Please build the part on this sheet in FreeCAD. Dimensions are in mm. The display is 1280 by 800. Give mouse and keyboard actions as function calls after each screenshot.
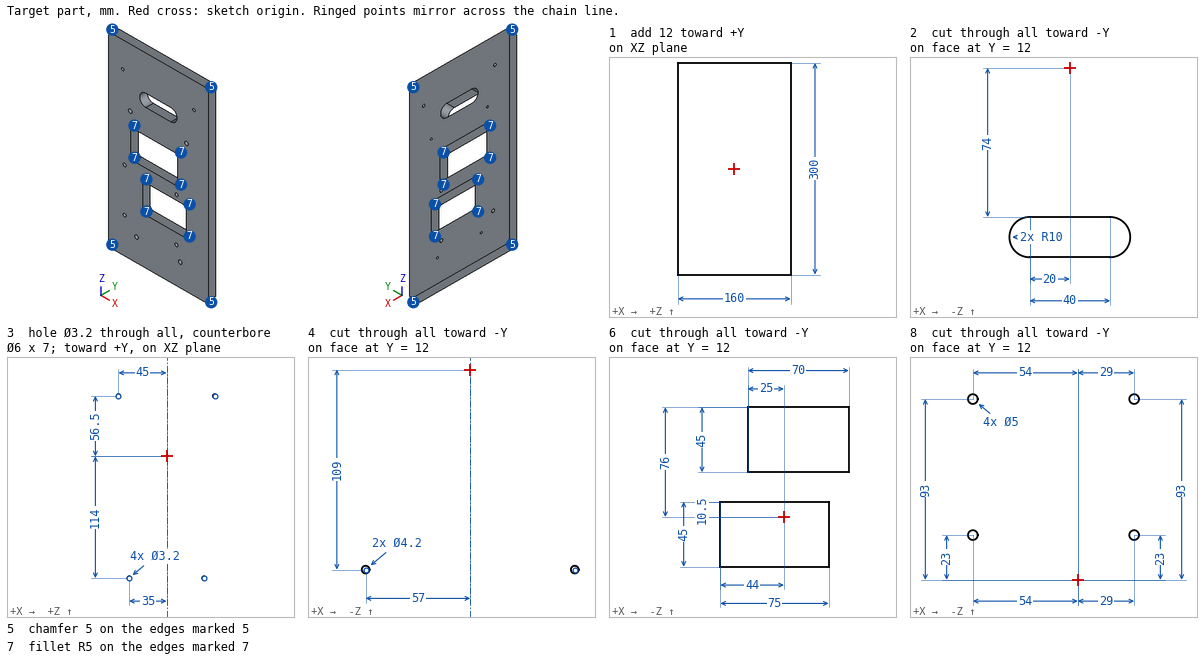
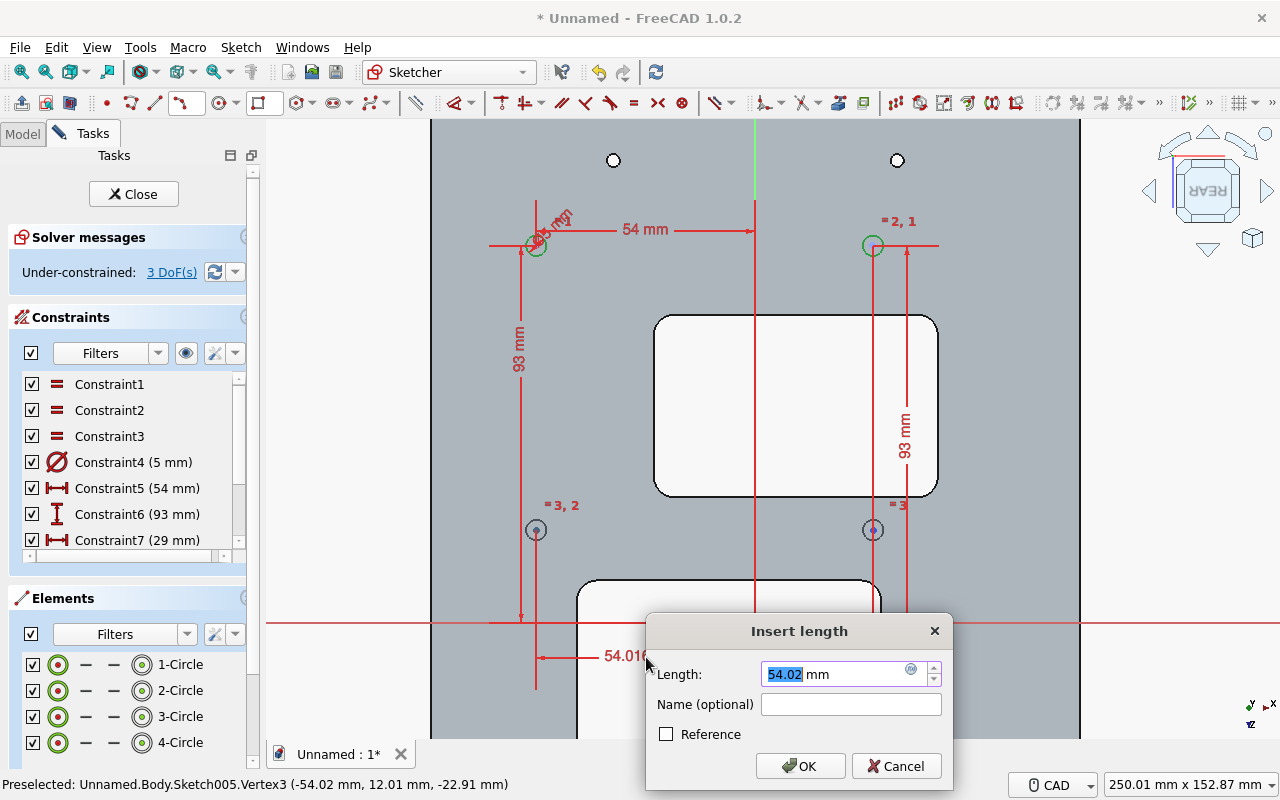
text(54)
key(Return)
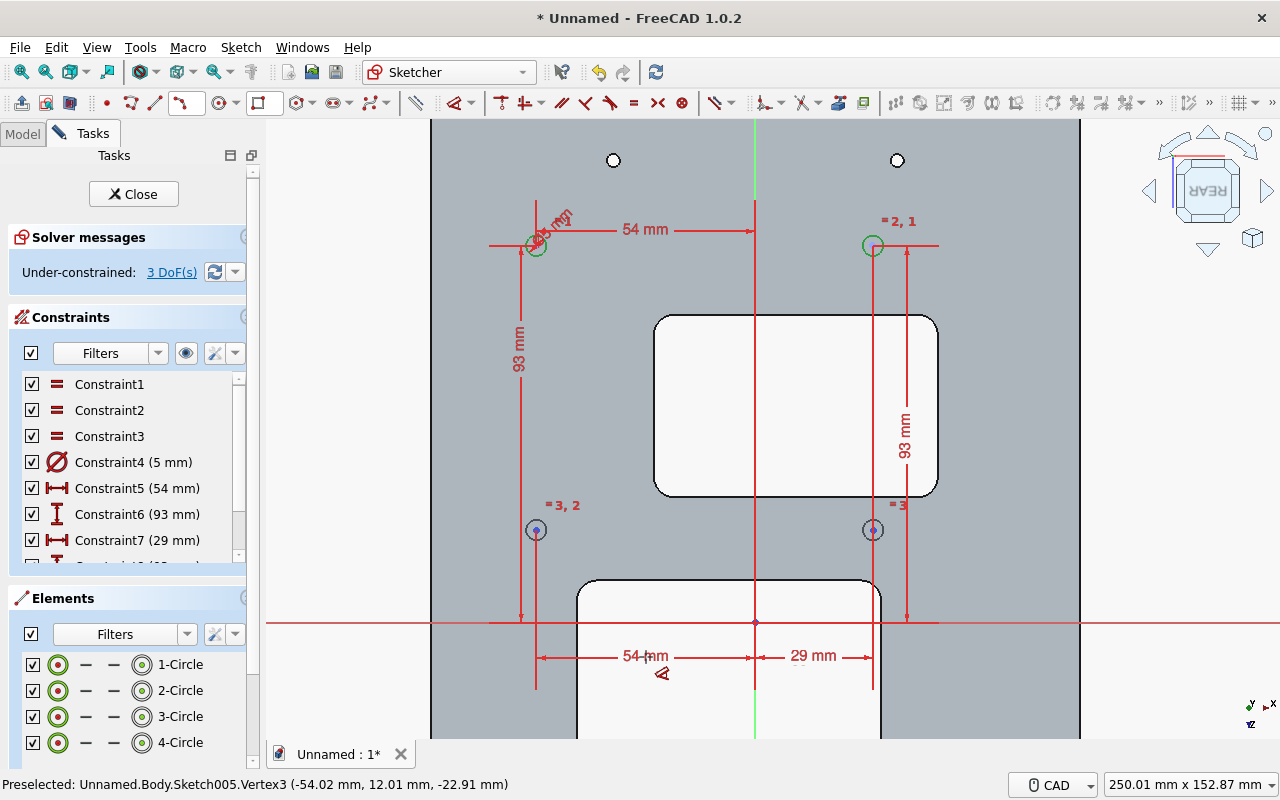
click(536, 530)
click(502, 577)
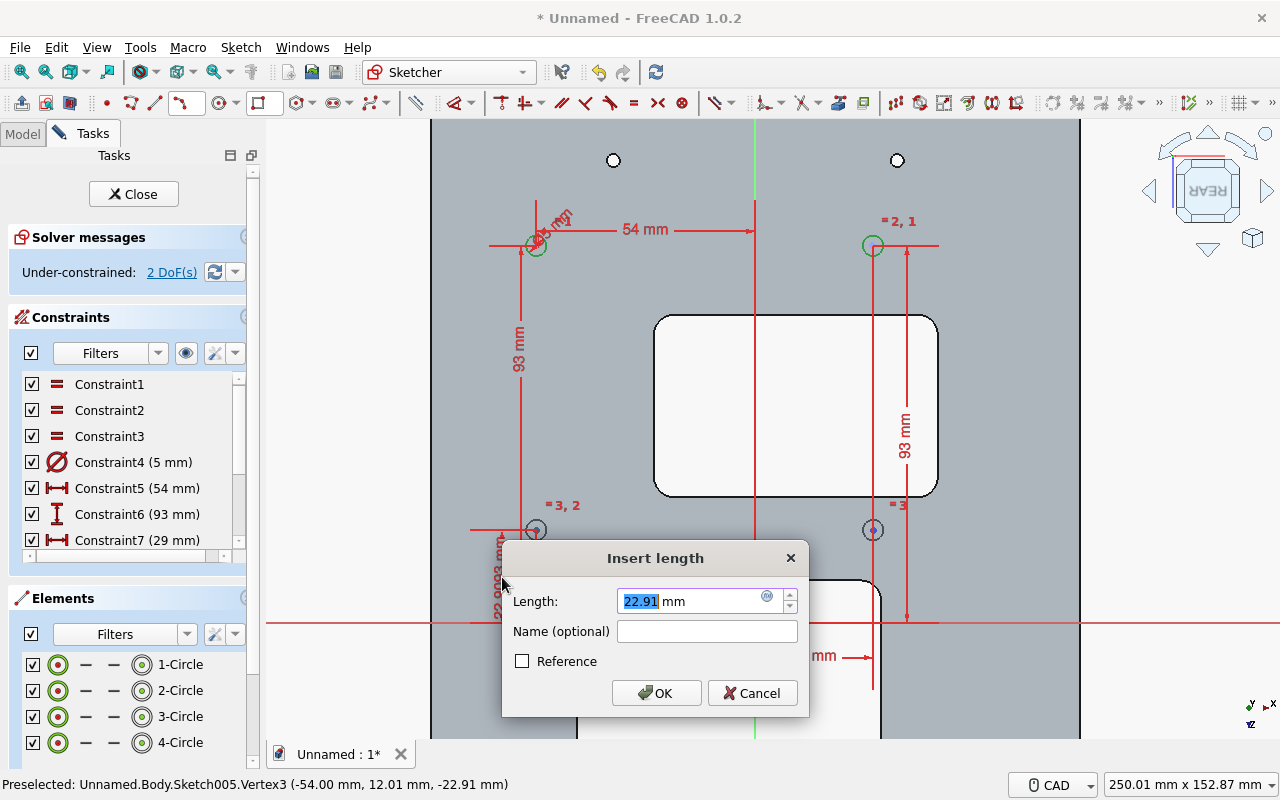
text(23)
key(Return)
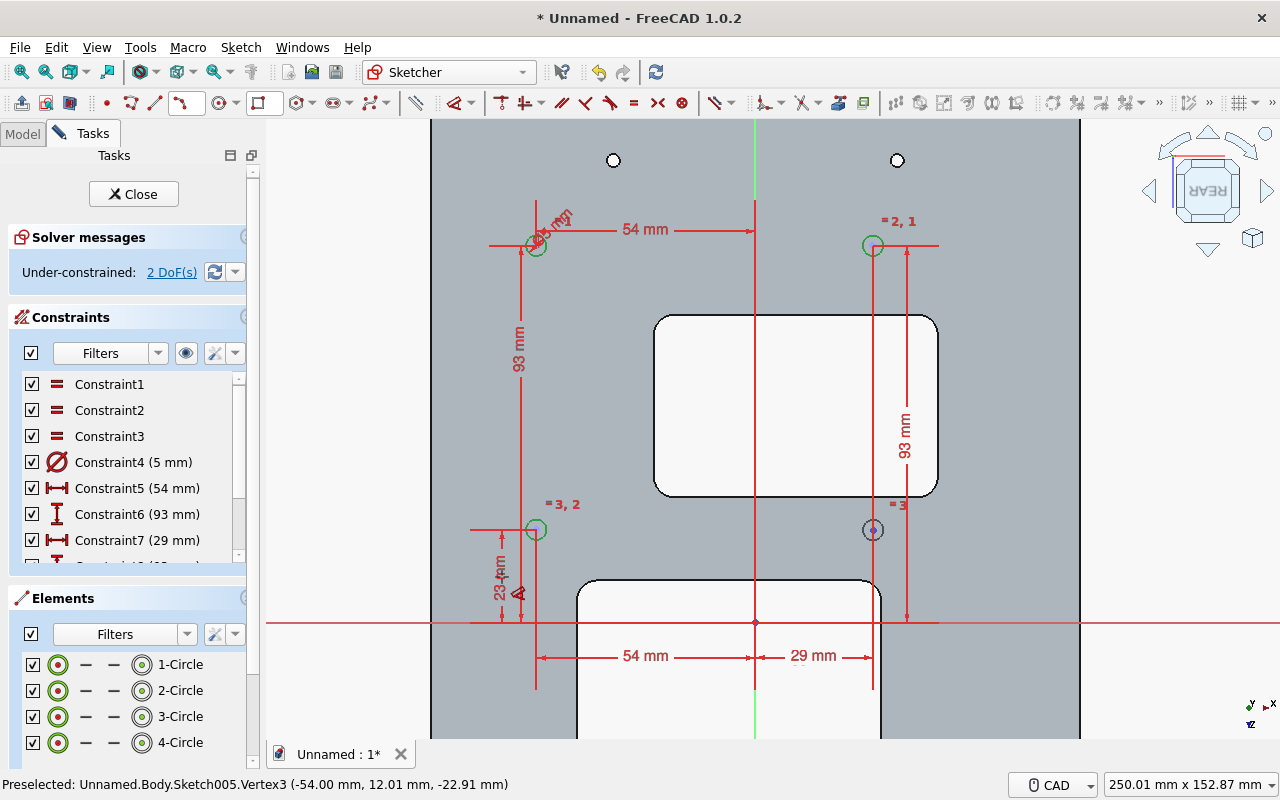
click(873, 530)
click(814, 496)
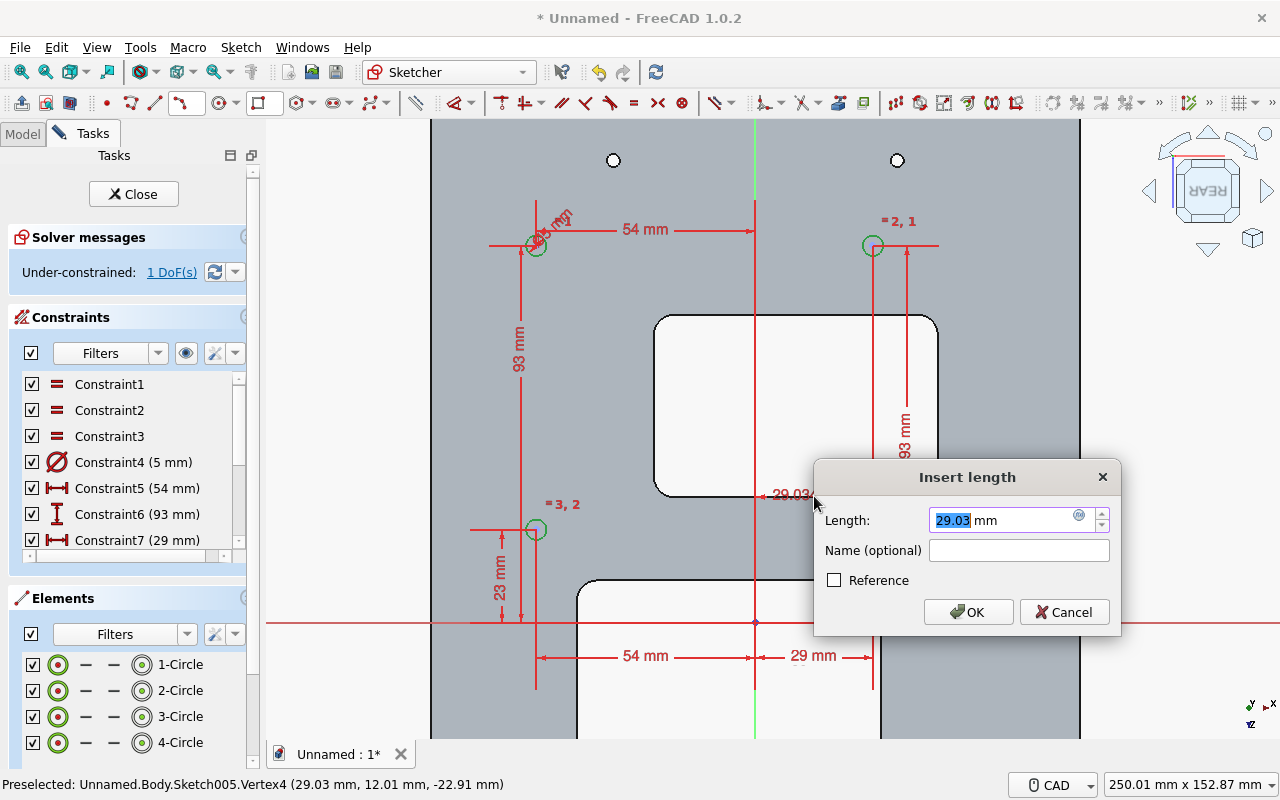
text(29)
key(Return)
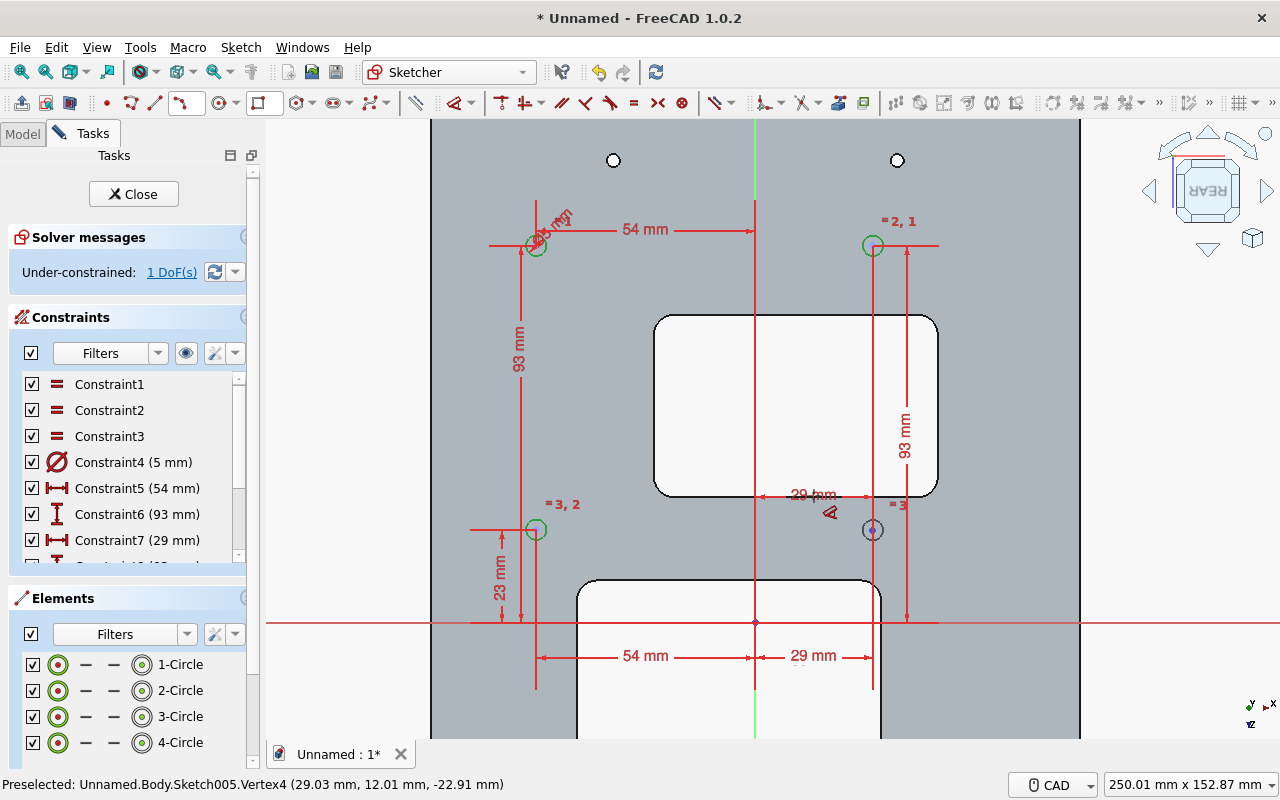
click(873, 530)
click(907, 577)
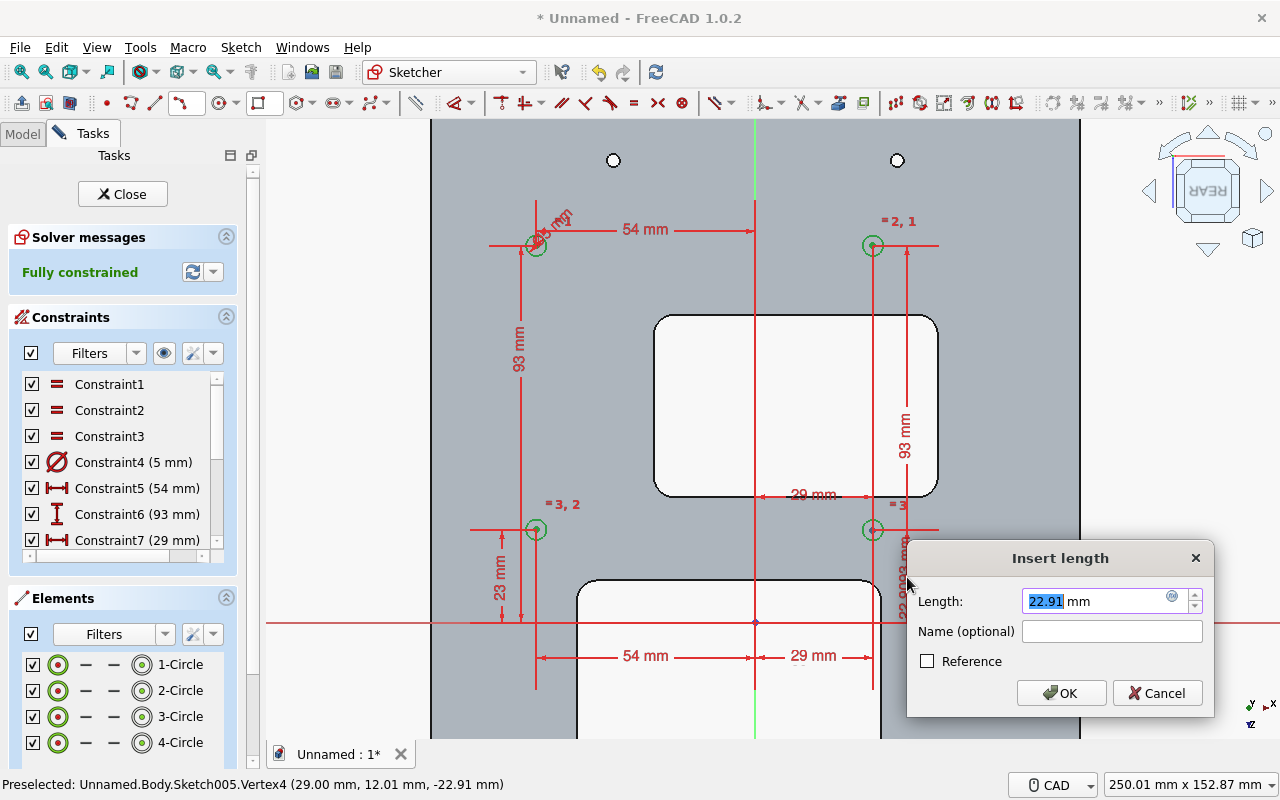
text(23)
key(Return)
key(Escape)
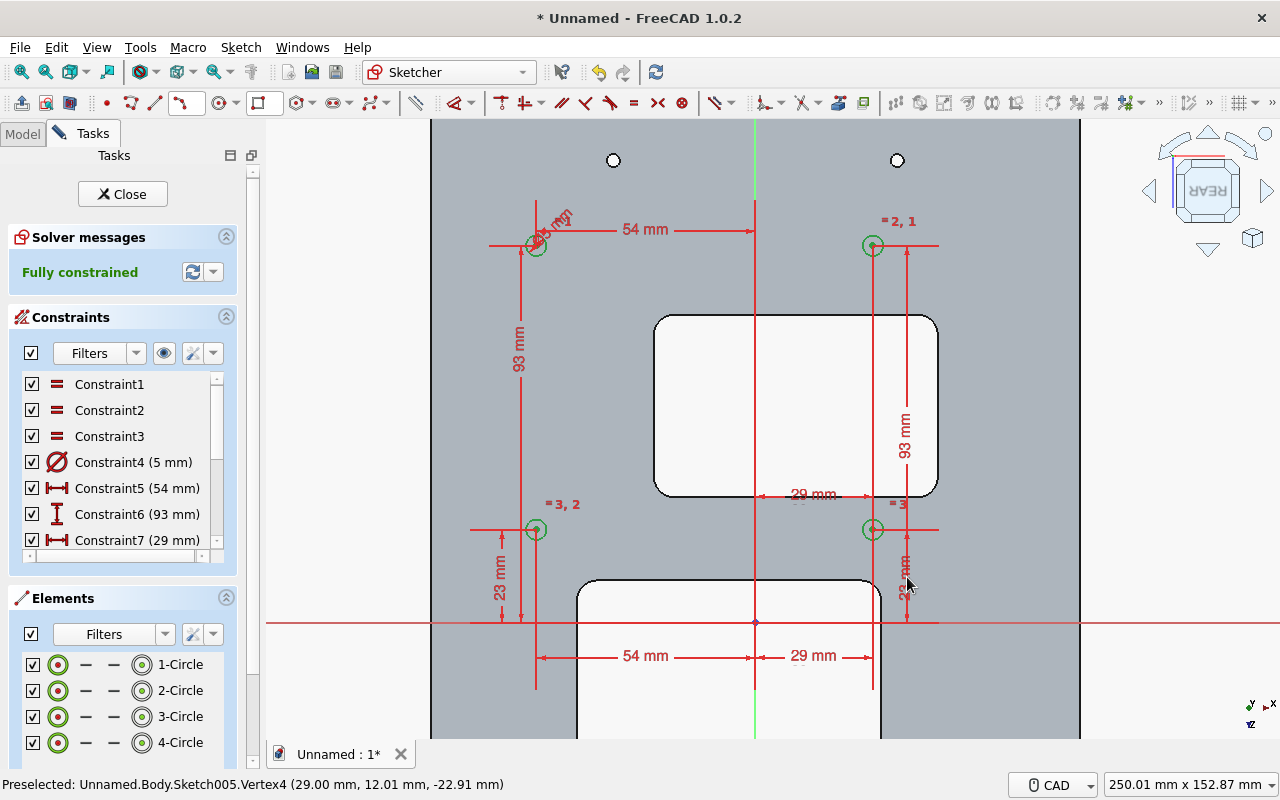
click(123, 194)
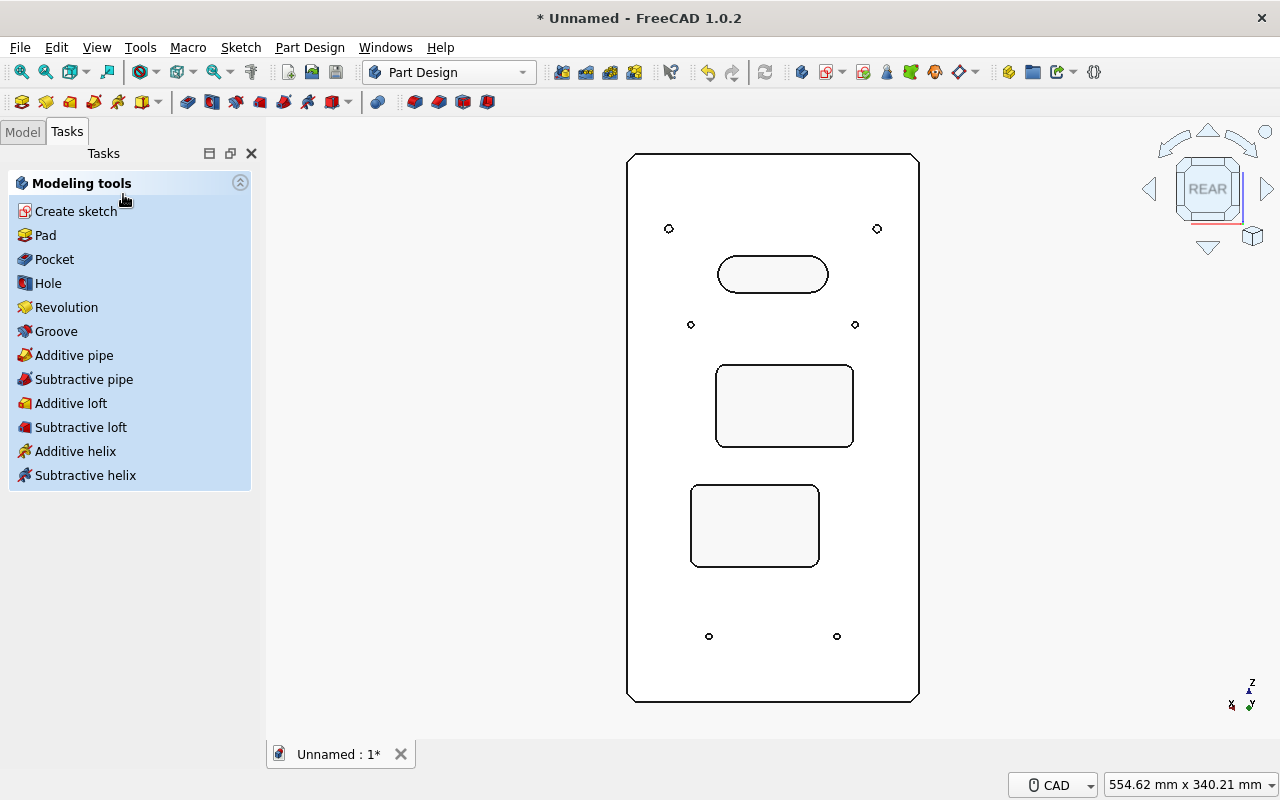
click(188, 102)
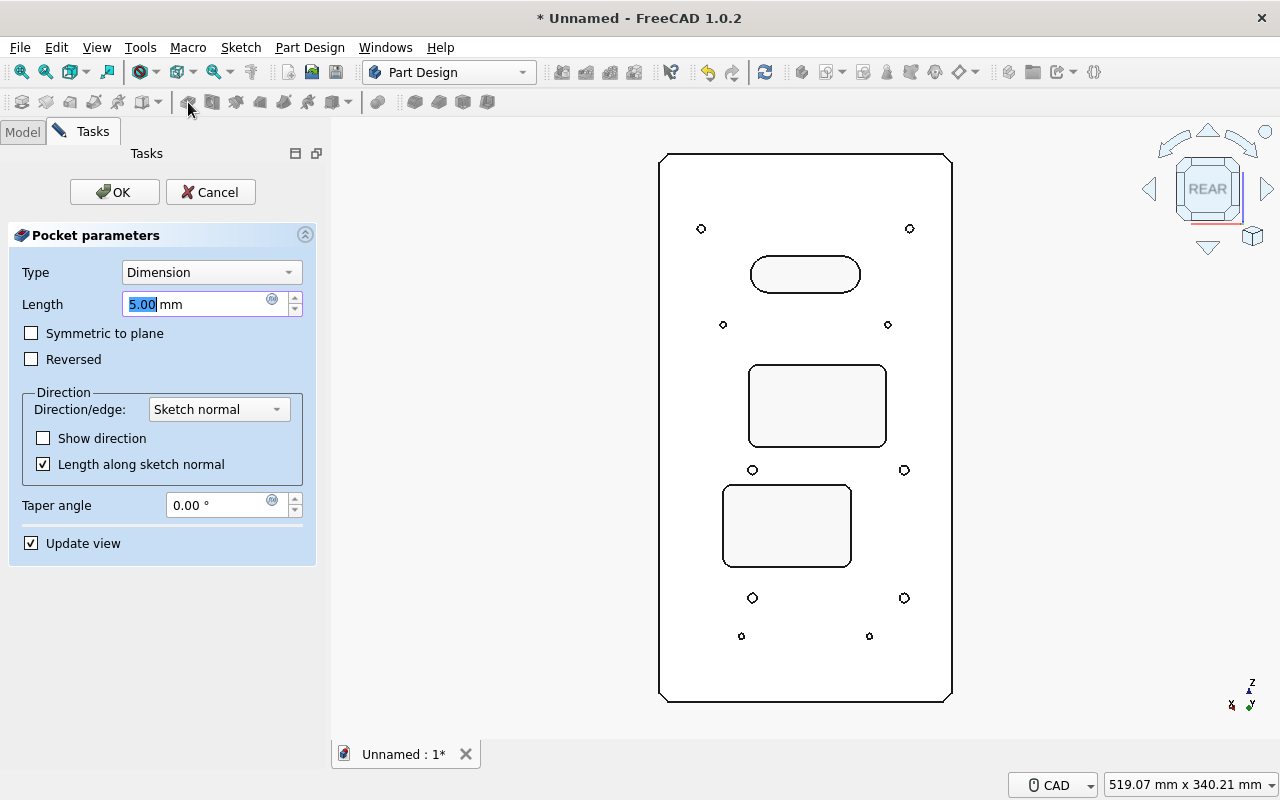
click(212, 272)